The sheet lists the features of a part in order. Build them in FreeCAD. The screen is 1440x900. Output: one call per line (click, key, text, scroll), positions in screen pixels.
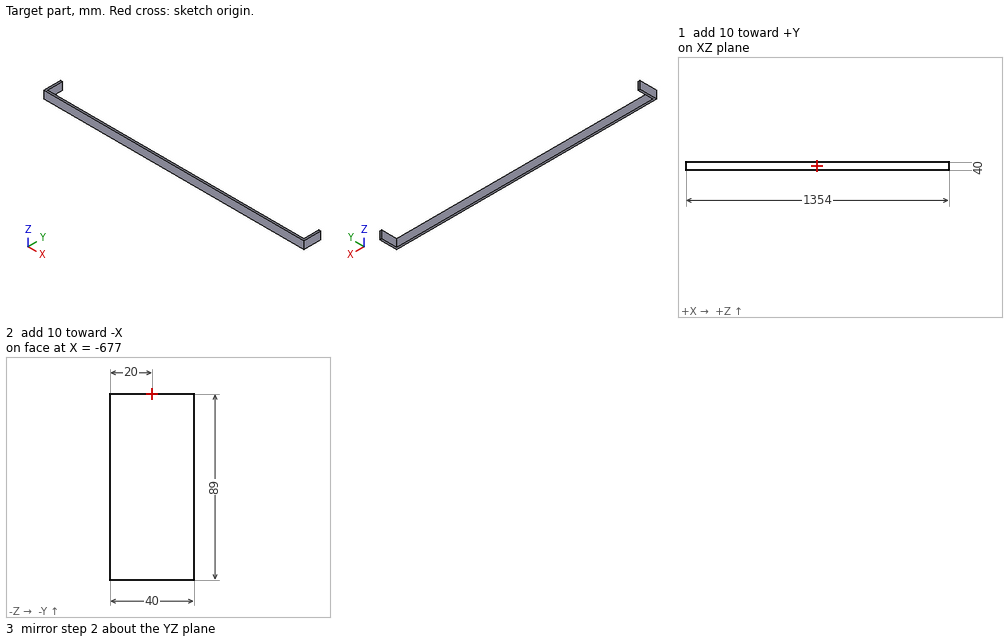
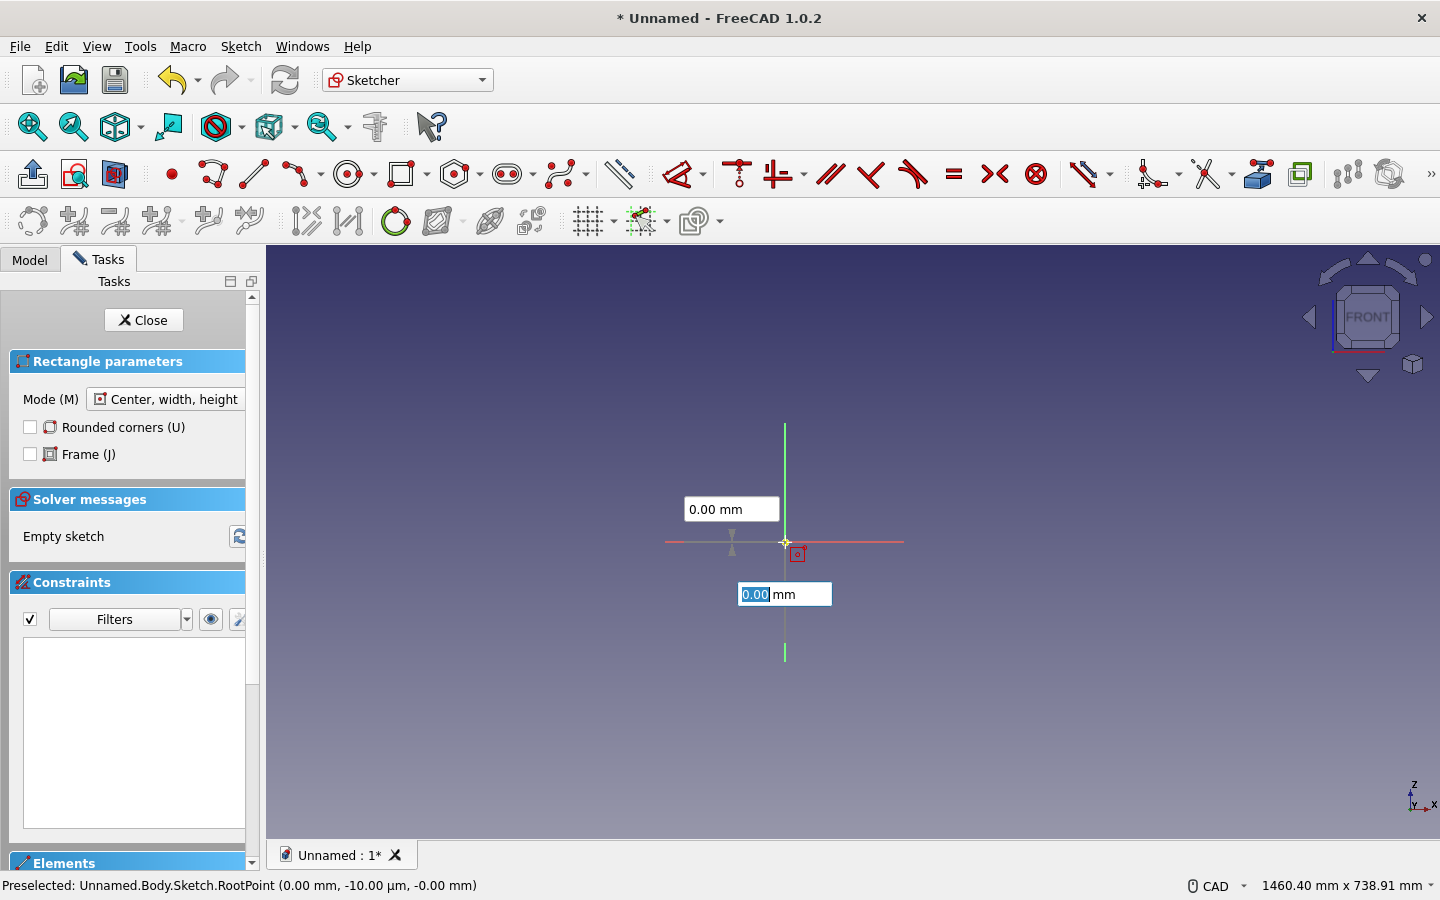
scroll(783, 541, down, 2)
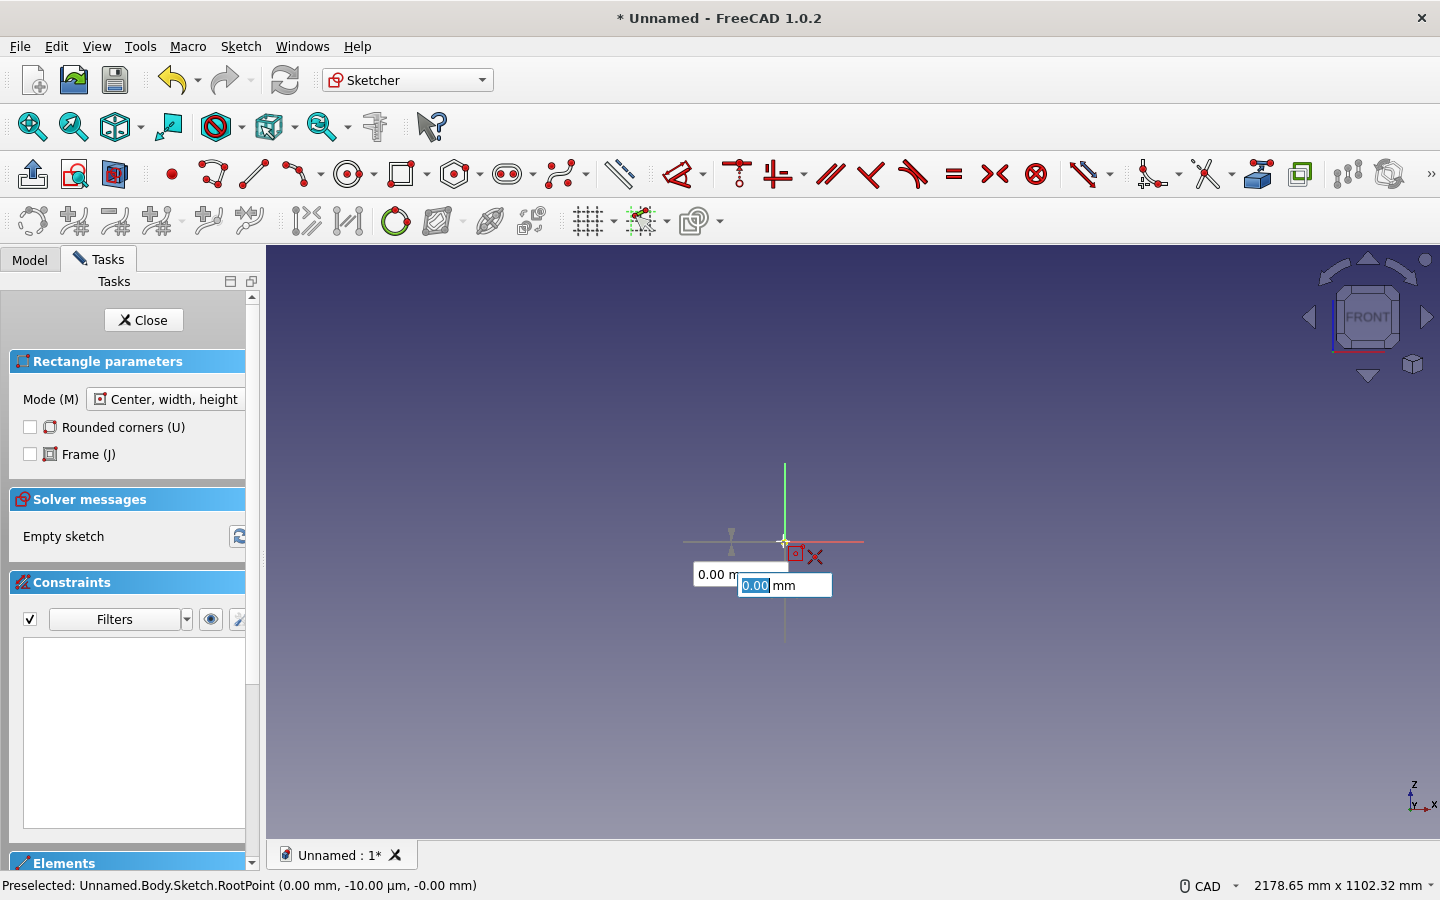
scroll(1149, 531, up, 2)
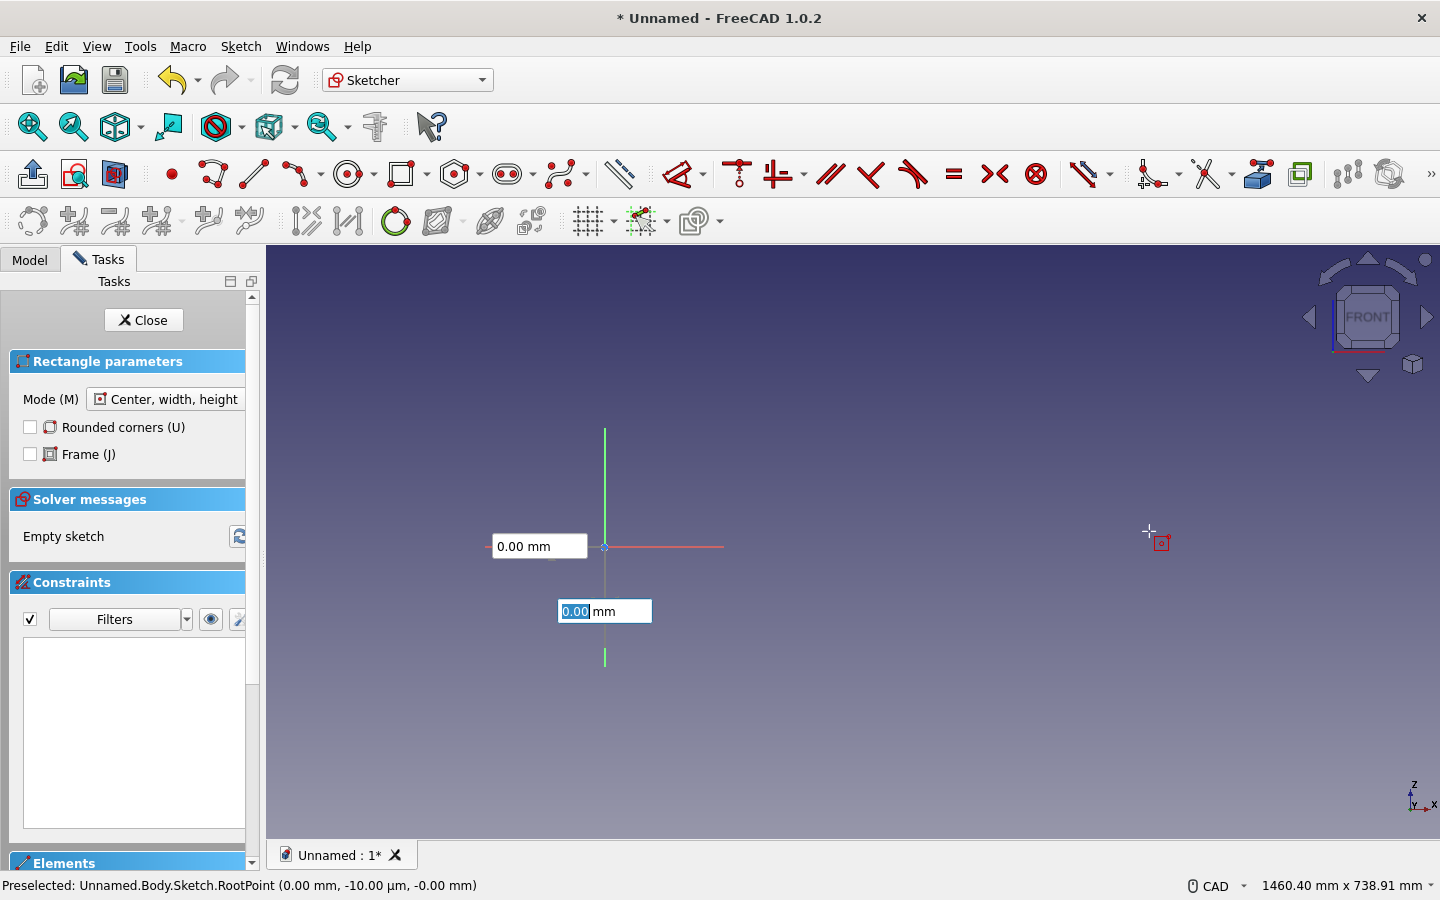
click(1149, 531)
key(Escape)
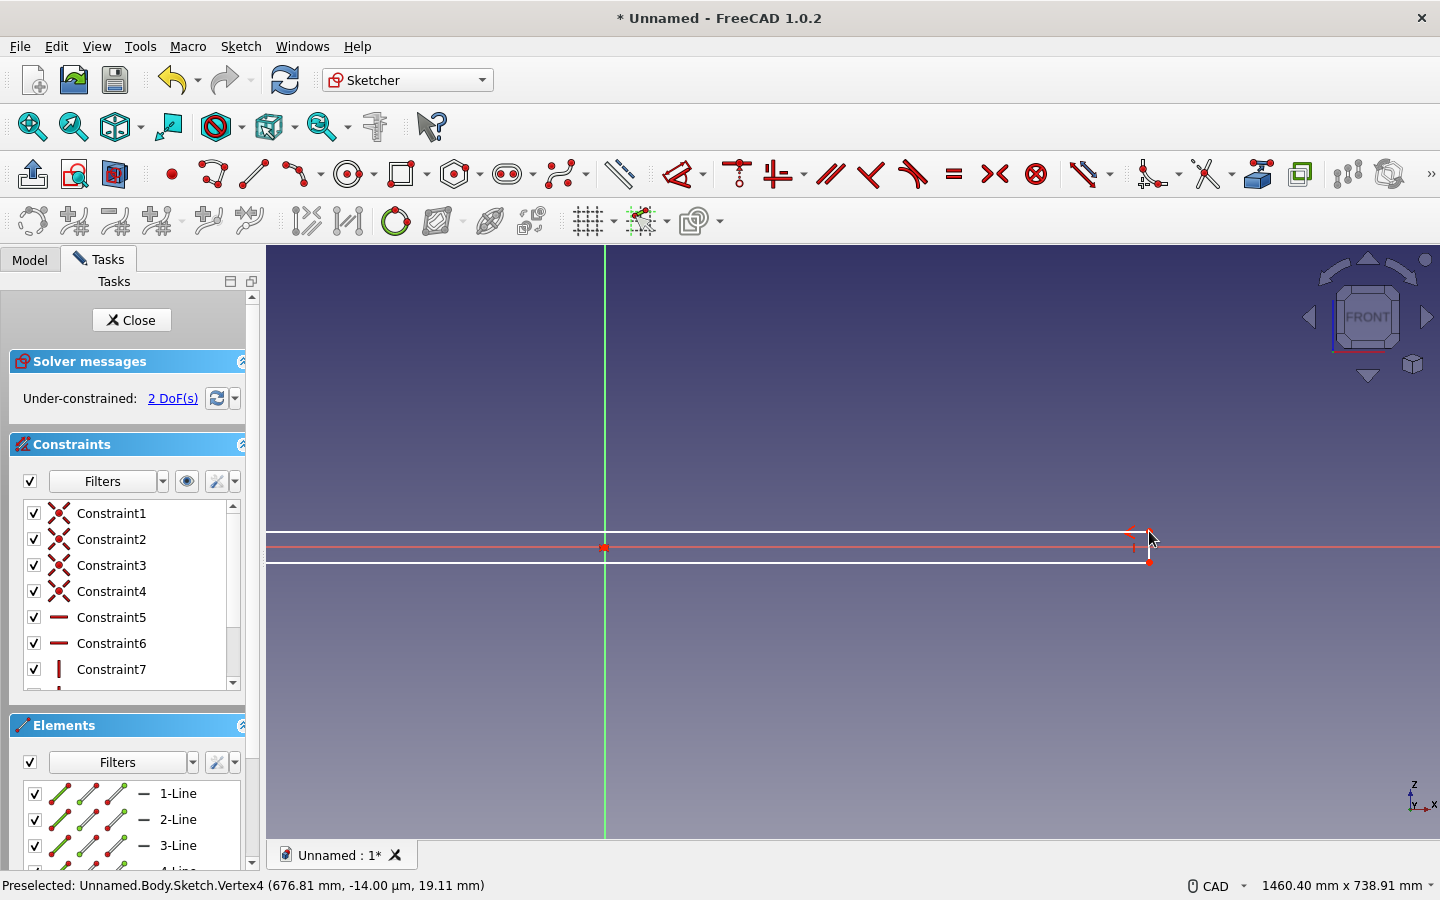
scroll(1149, 550, up, 2)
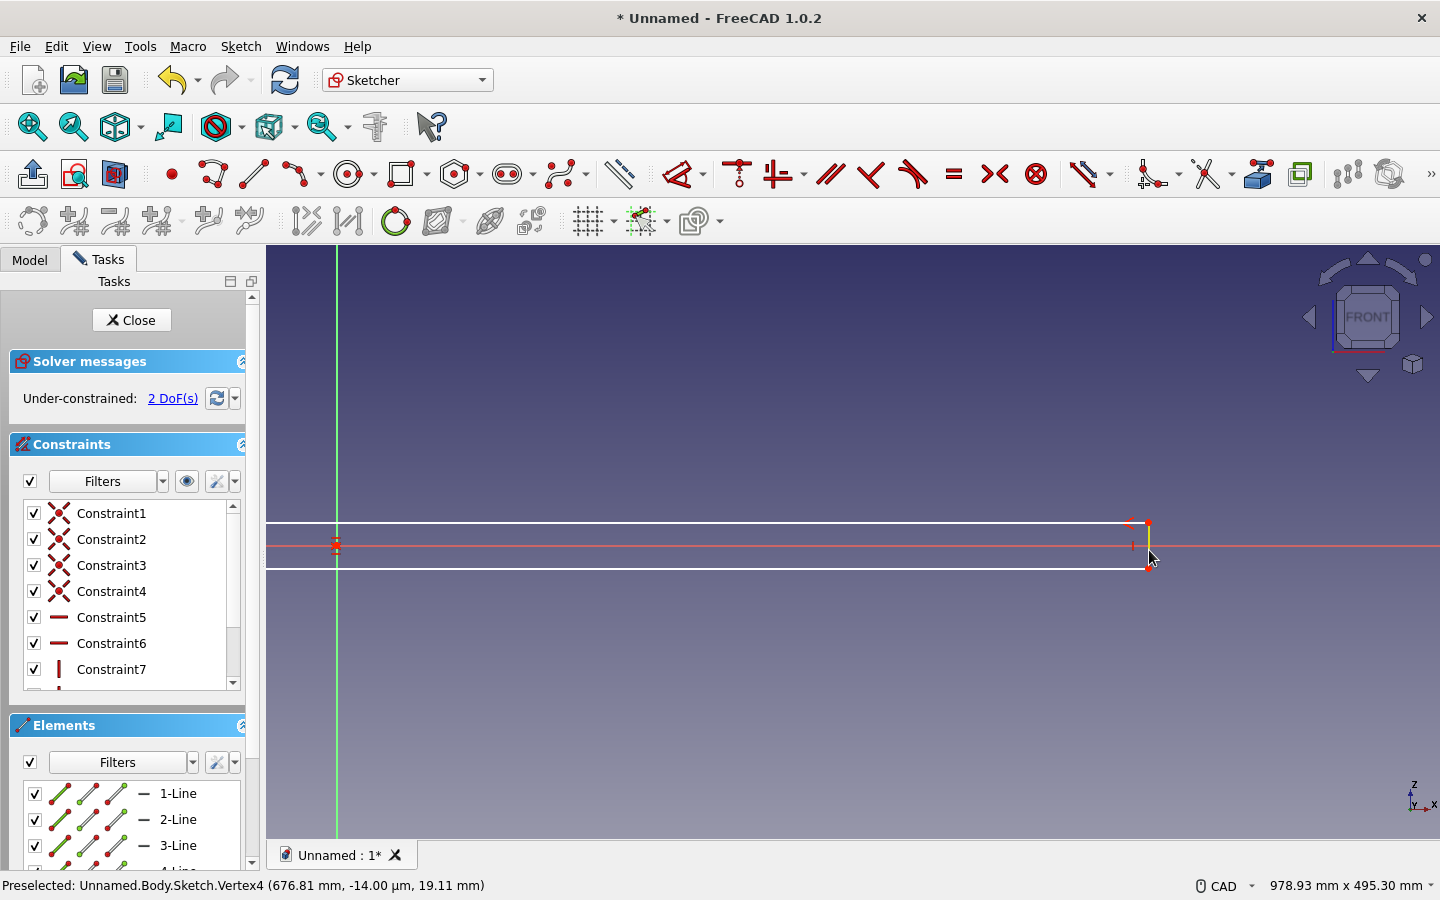
click(1149, 550)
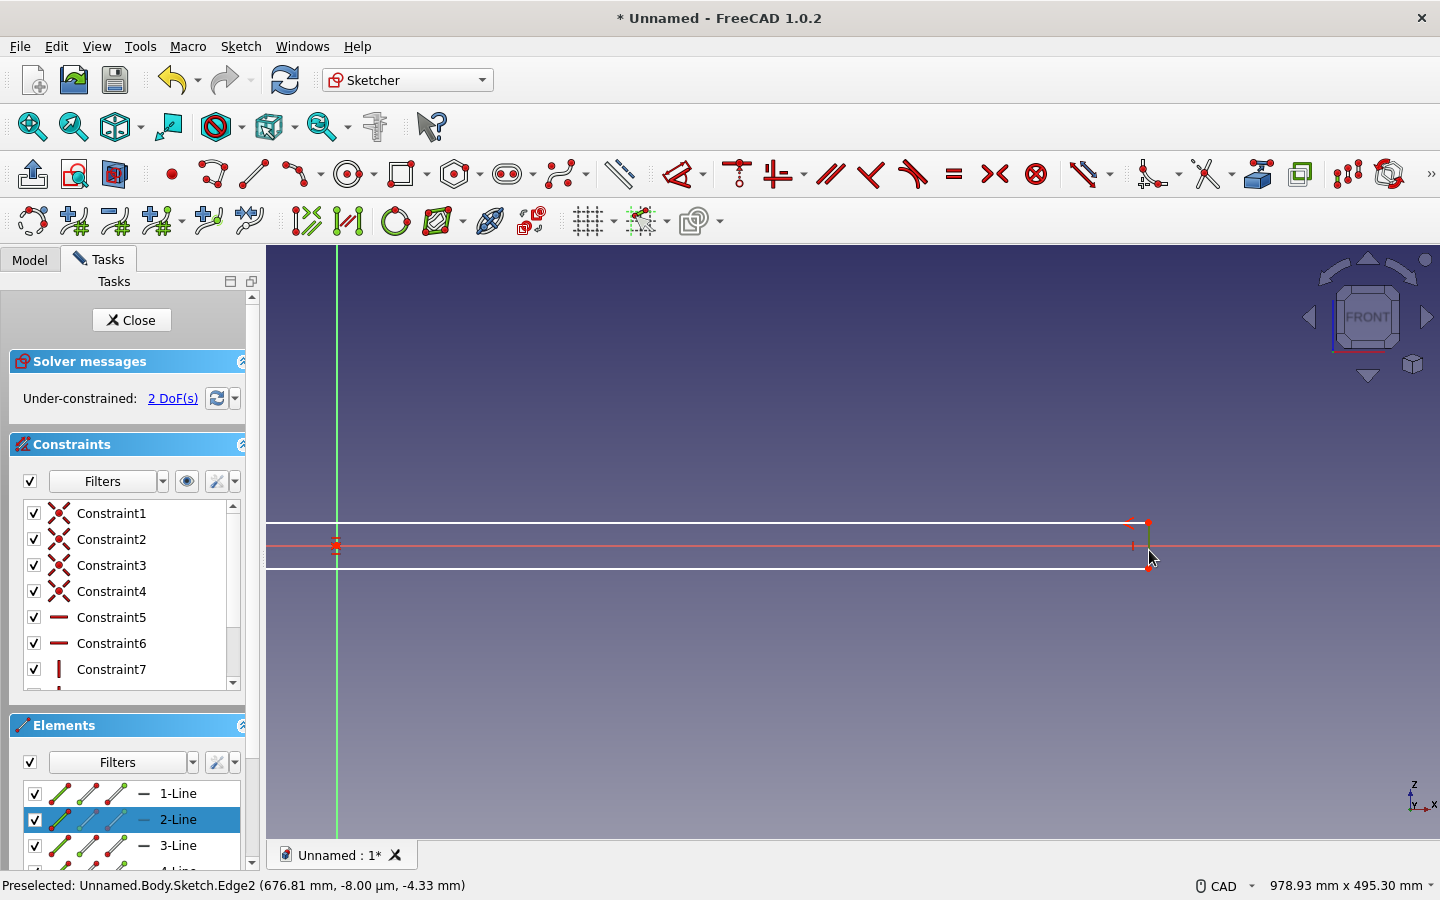
click(702, 174)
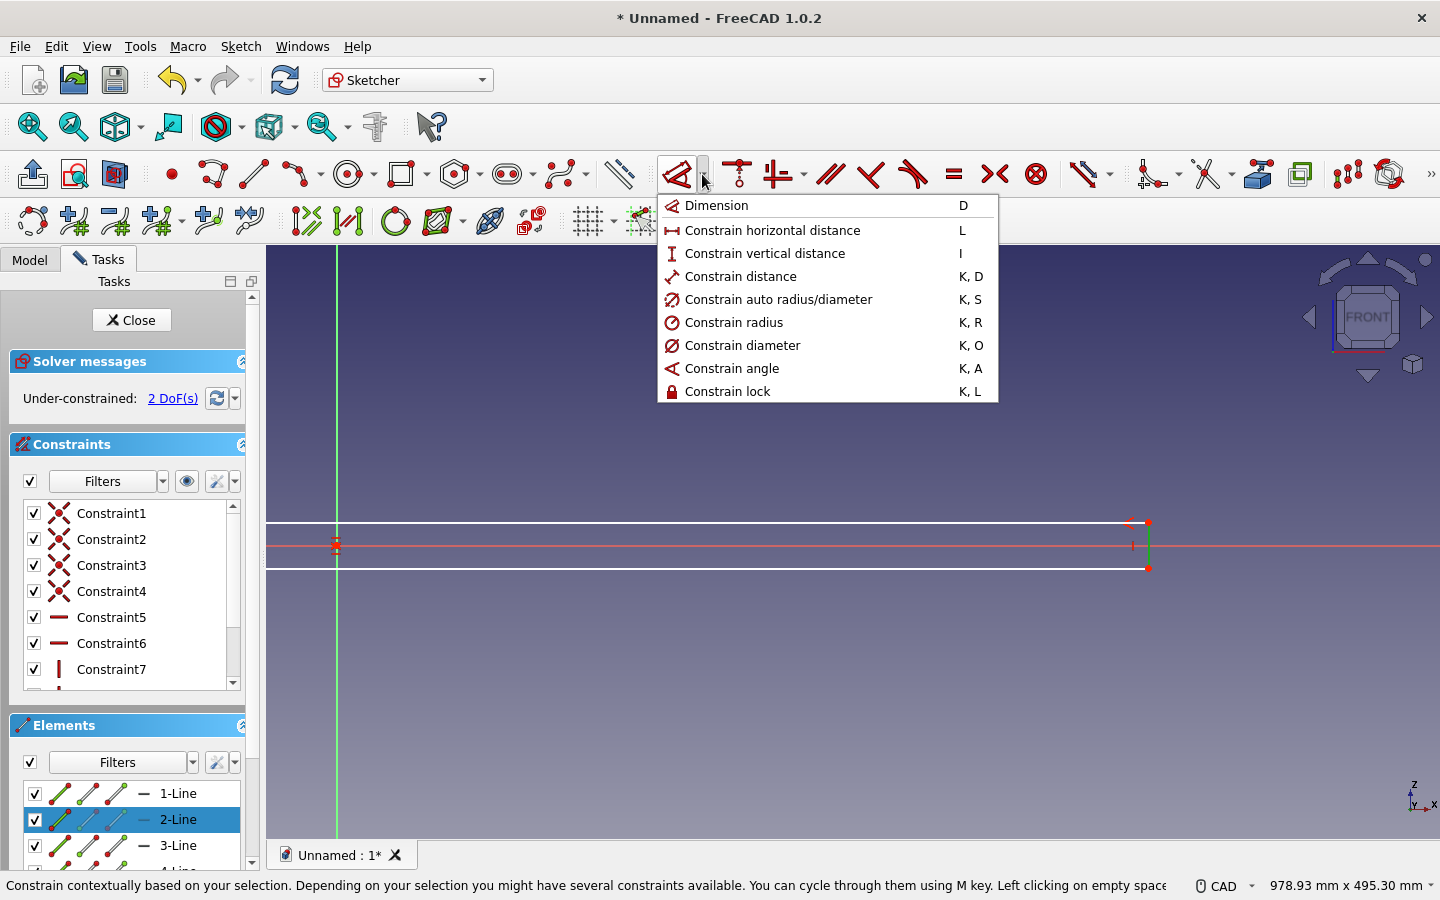
click(828, 254)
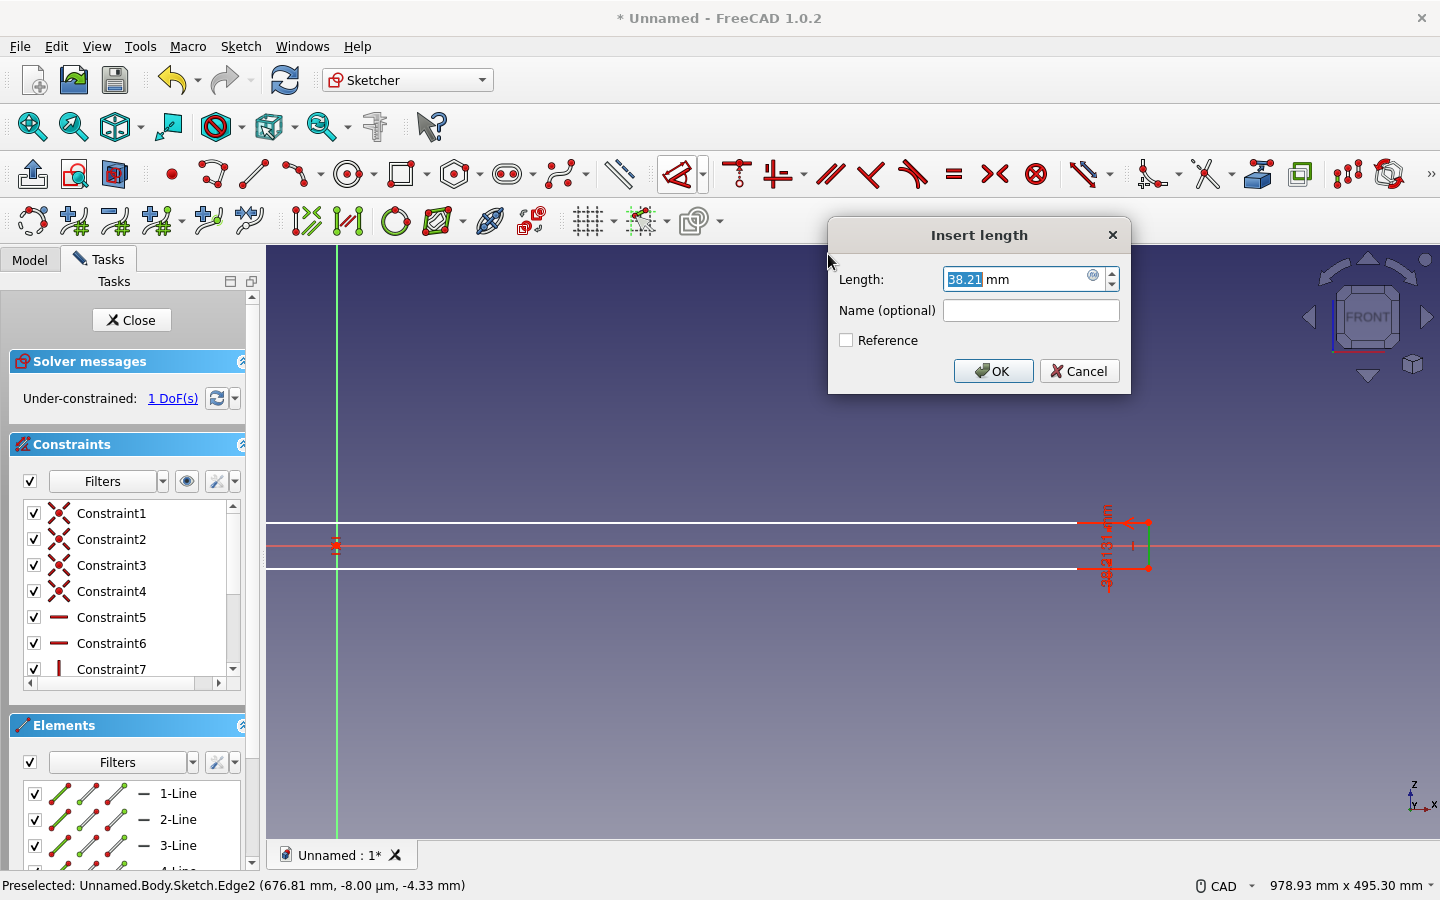
text(40)
key(Return)